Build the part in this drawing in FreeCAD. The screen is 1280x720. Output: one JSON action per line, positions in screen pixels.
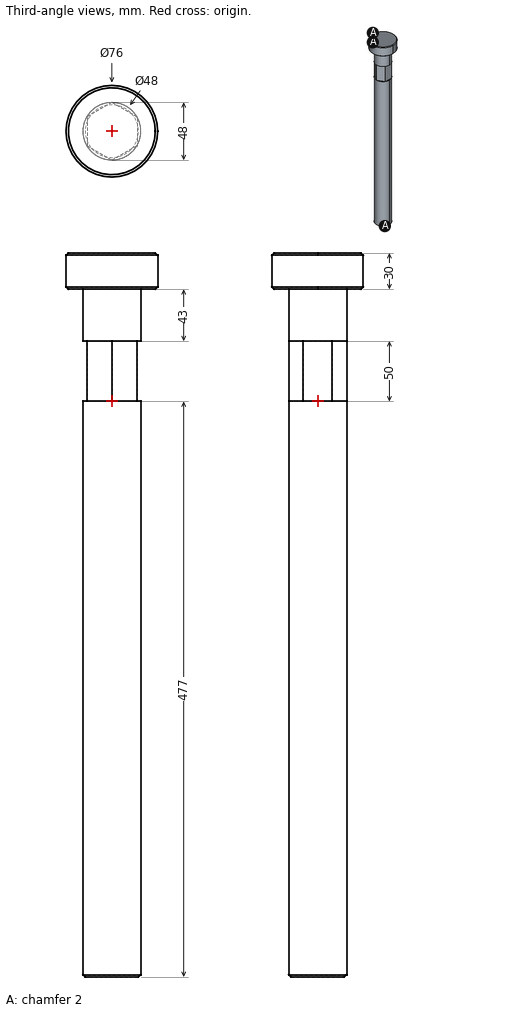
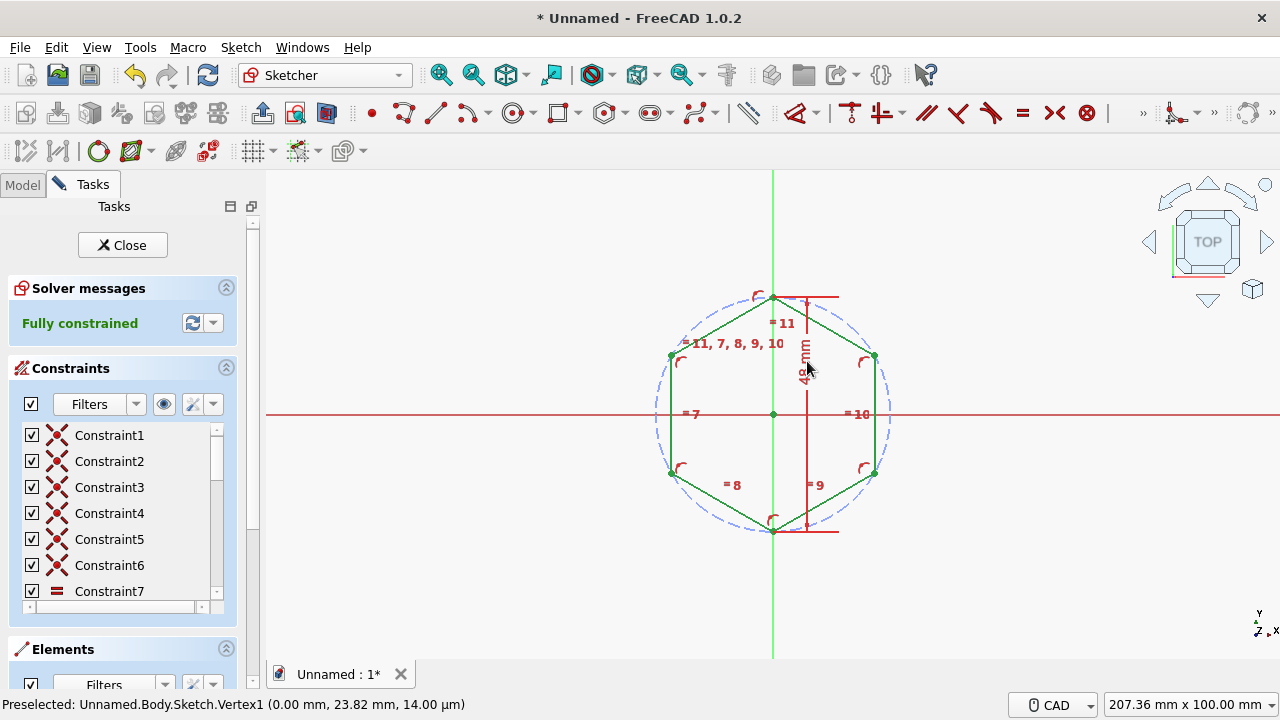
{"action": "left_click", "coordinate": [123, 245]}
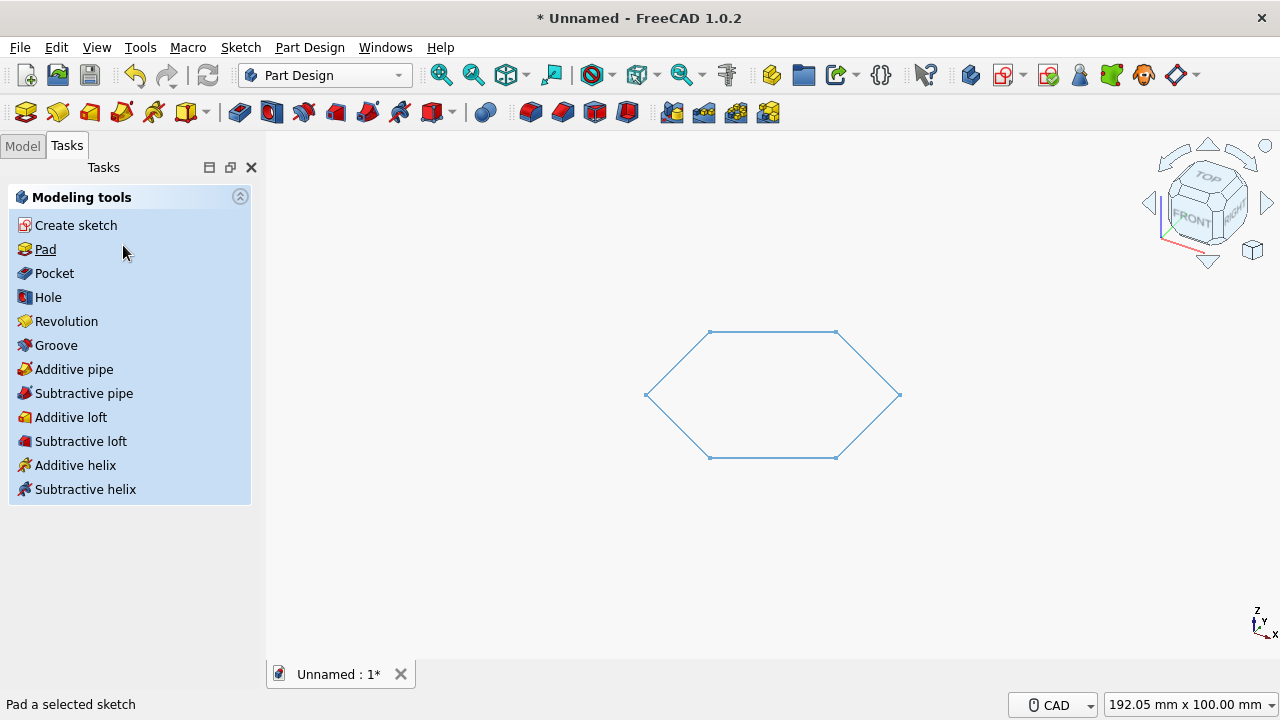
{"action": "left_click", "coordinate": [26, 112]}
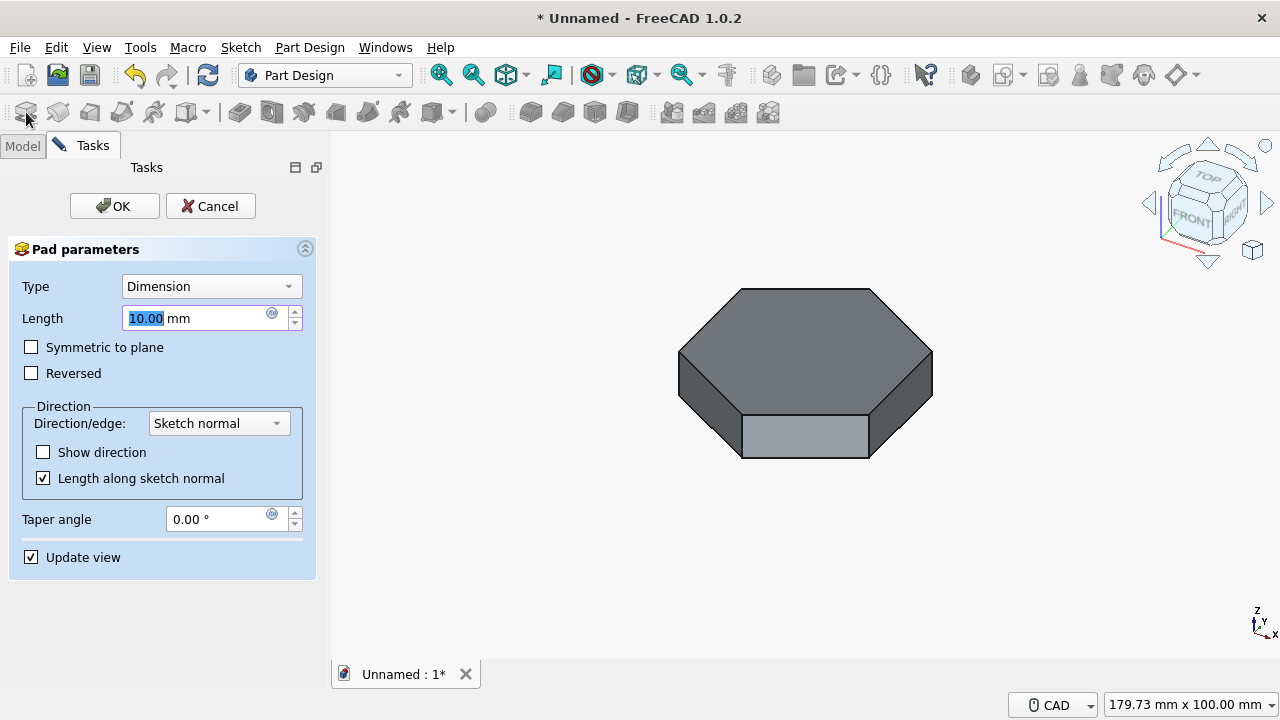
{"action": "type", "text": "50"}
{"action": "key", "text": "Tab"}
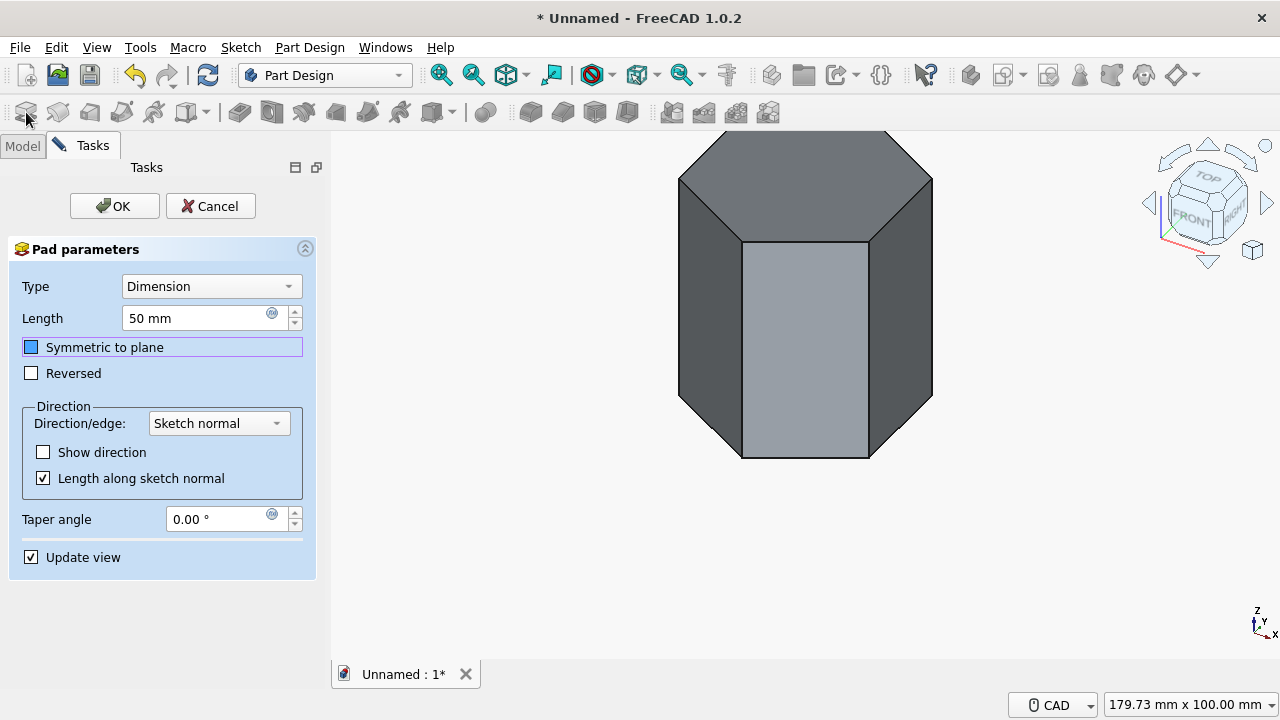
{"action": "left_click", "coordinate": [115, 206]}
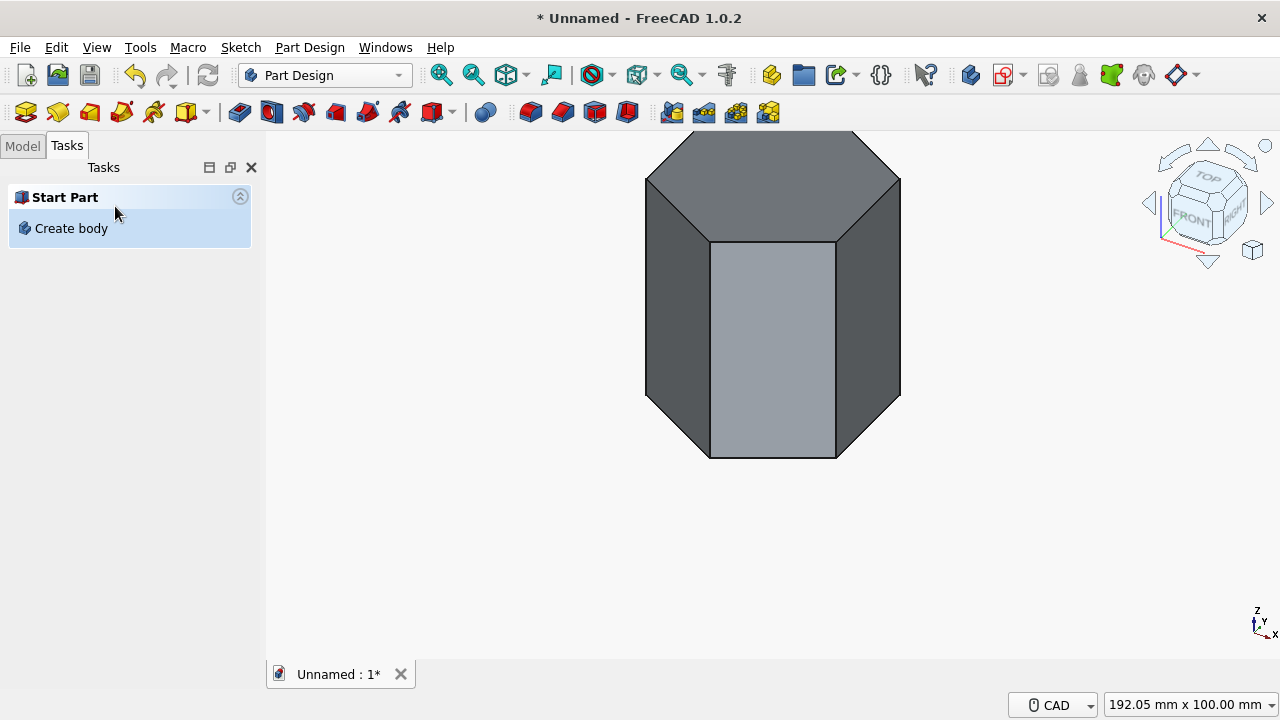
{"action": "left_click", "coordinate": [442, 76]}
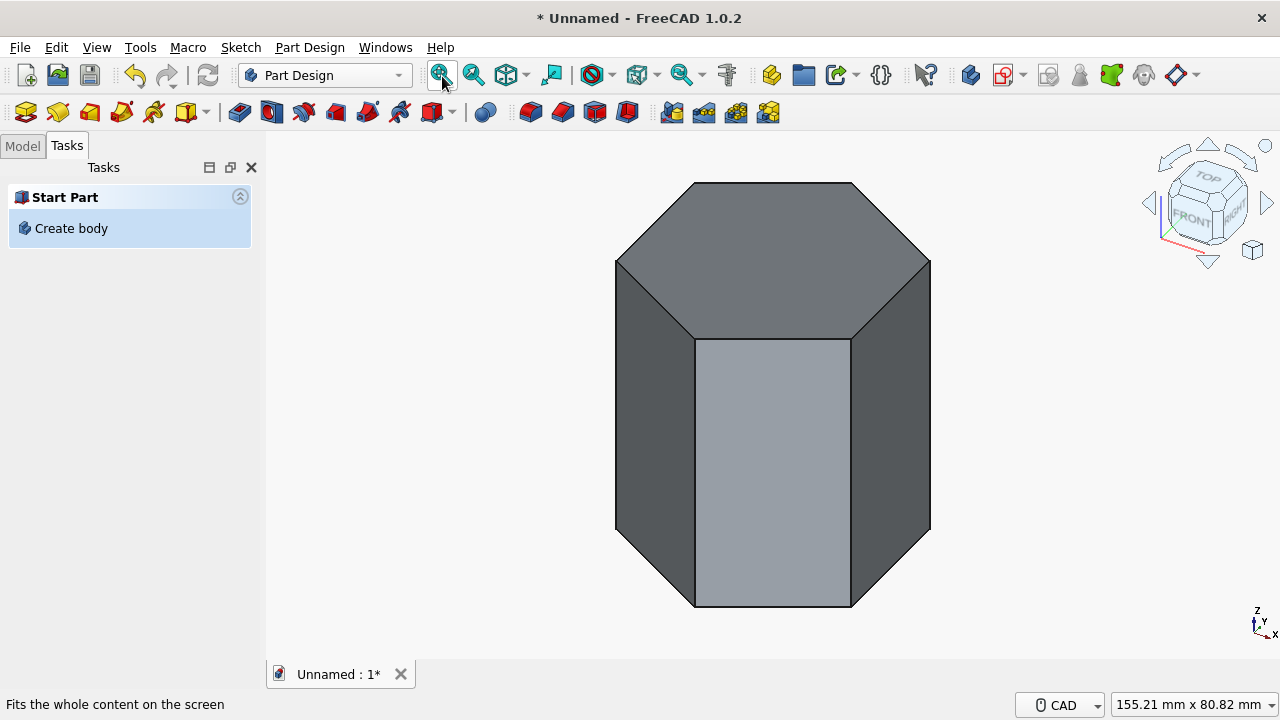
{"action": "left_click", "coordinate": [773, 260]}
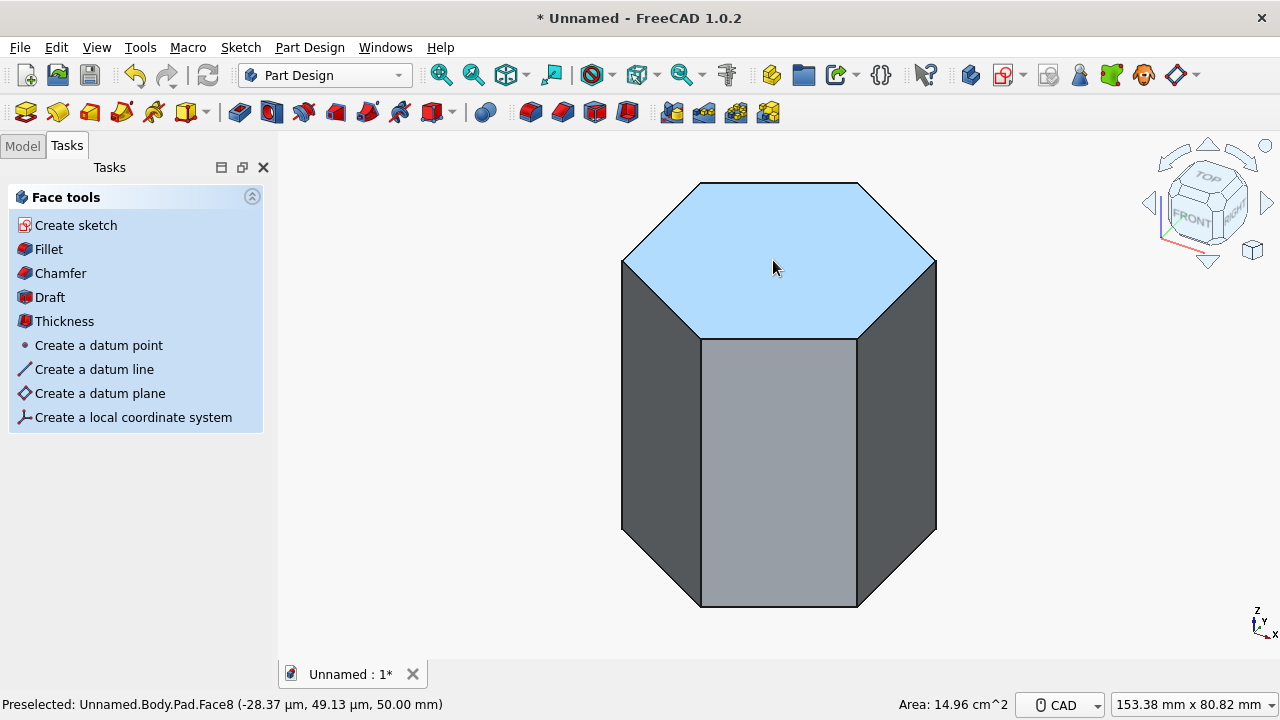
{"action": "left_click", "coordinate": [1004, 76]}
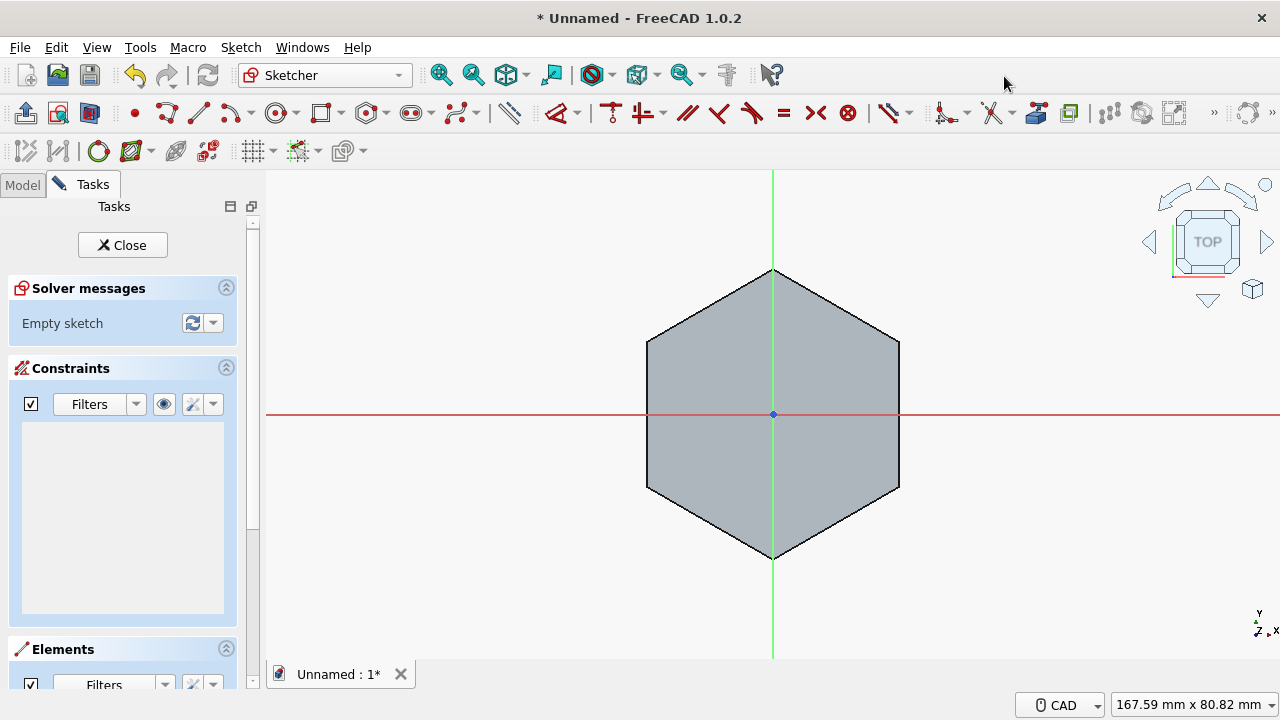
{"action": "left_click", "coordinate": [276, 114]}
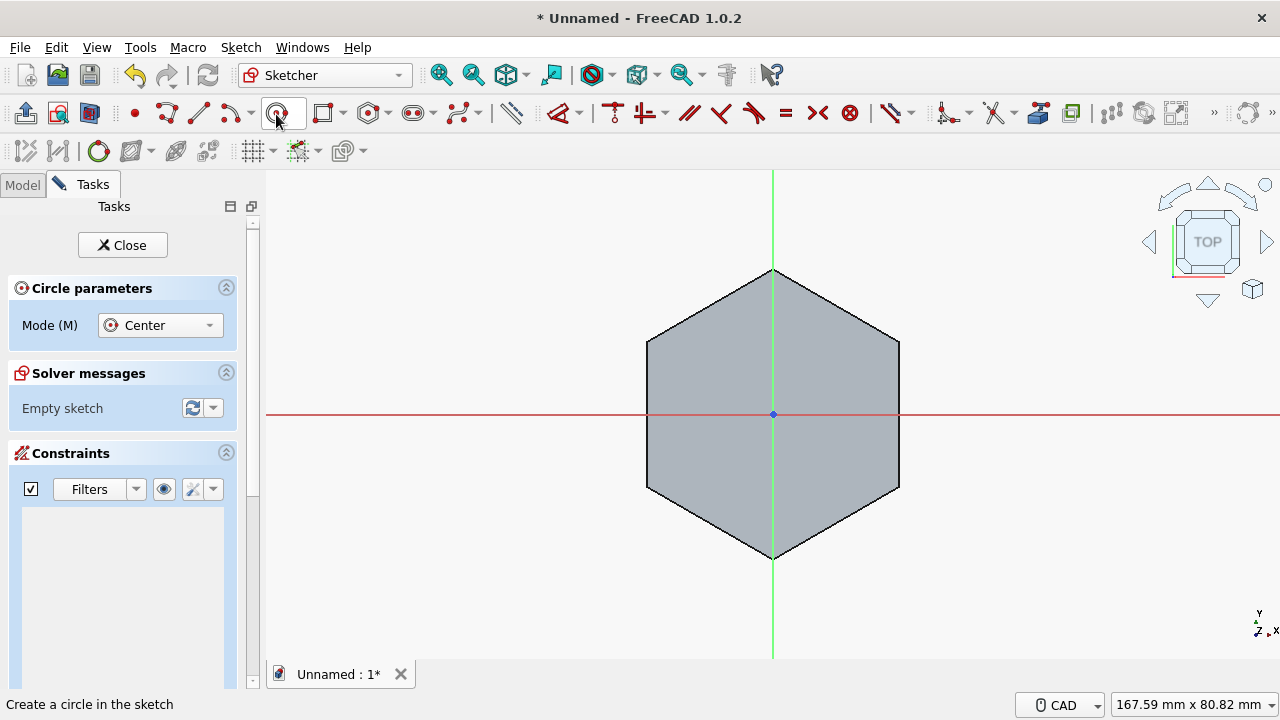
{"action": "left_click", "coordinate": [773, 414]}
{"action": "left_click", "coordinate": [876, 312]}
{"action": "key", "text": "Escape"}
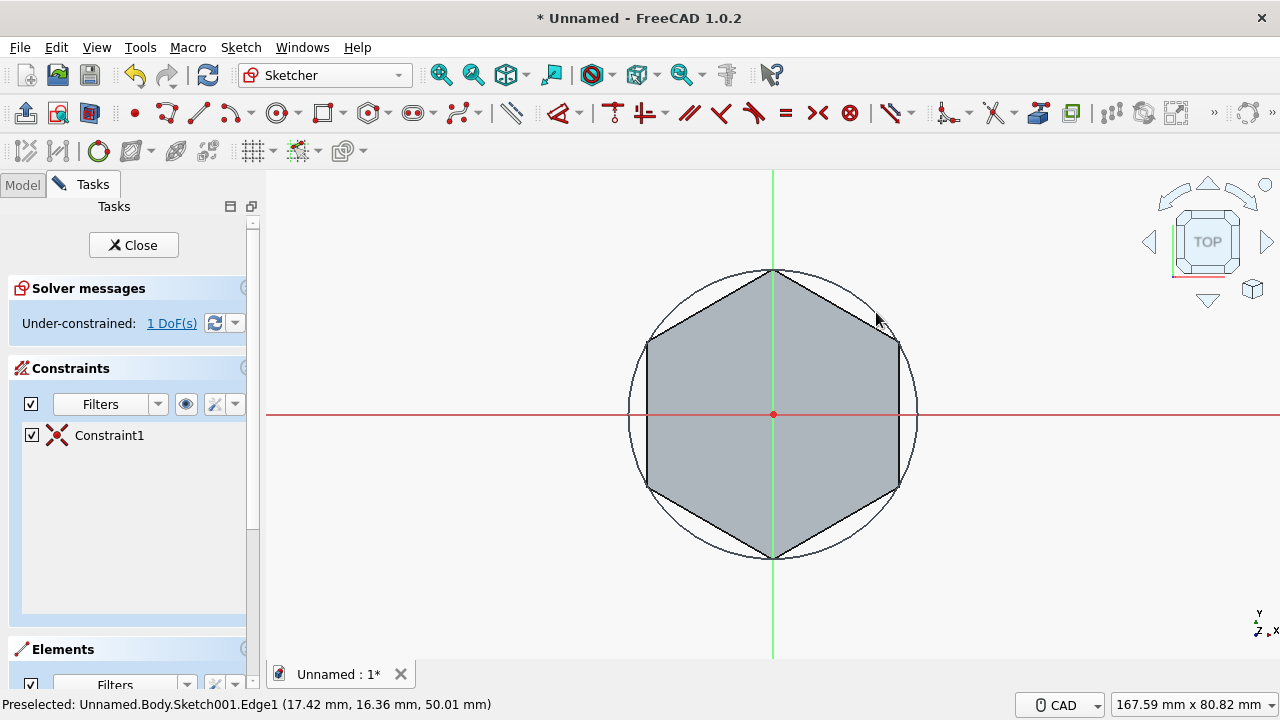
{"action": "left_click", "coordinate": [558, 114]}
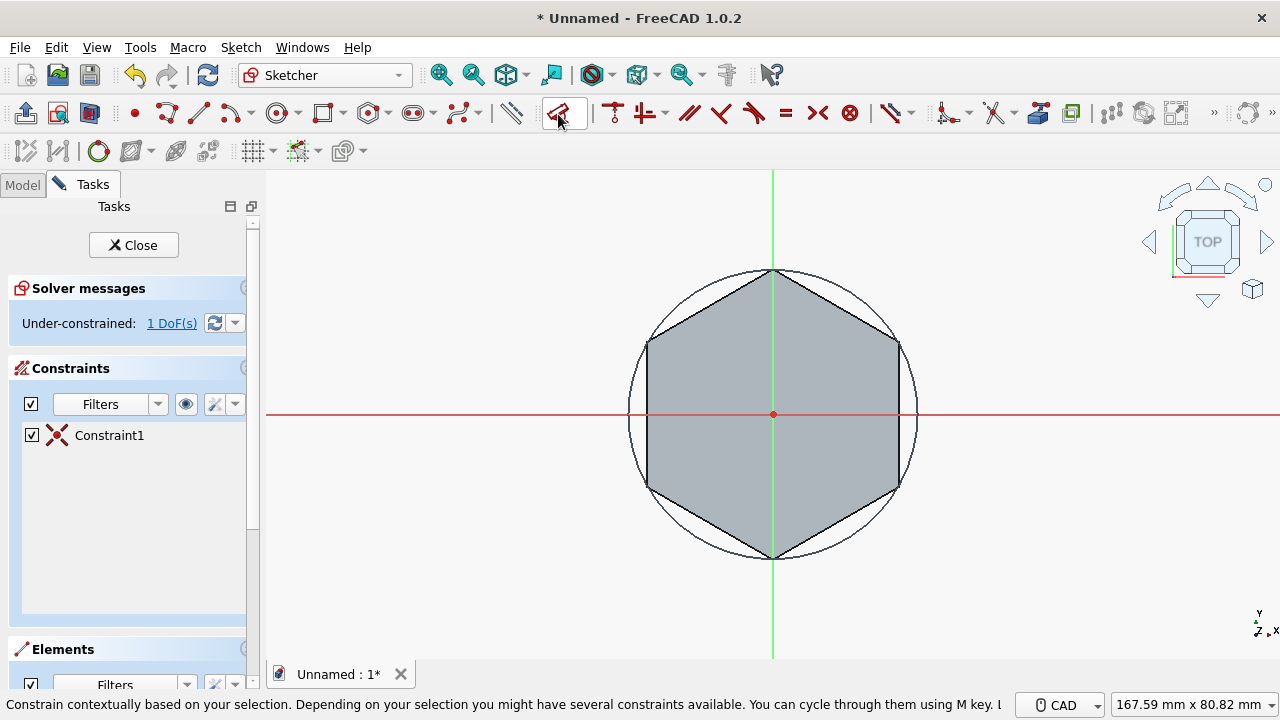
{"action": "left_click", "coordinate": [875, 312]}
{"action": "left_click", "coordinate": [898, 289]}